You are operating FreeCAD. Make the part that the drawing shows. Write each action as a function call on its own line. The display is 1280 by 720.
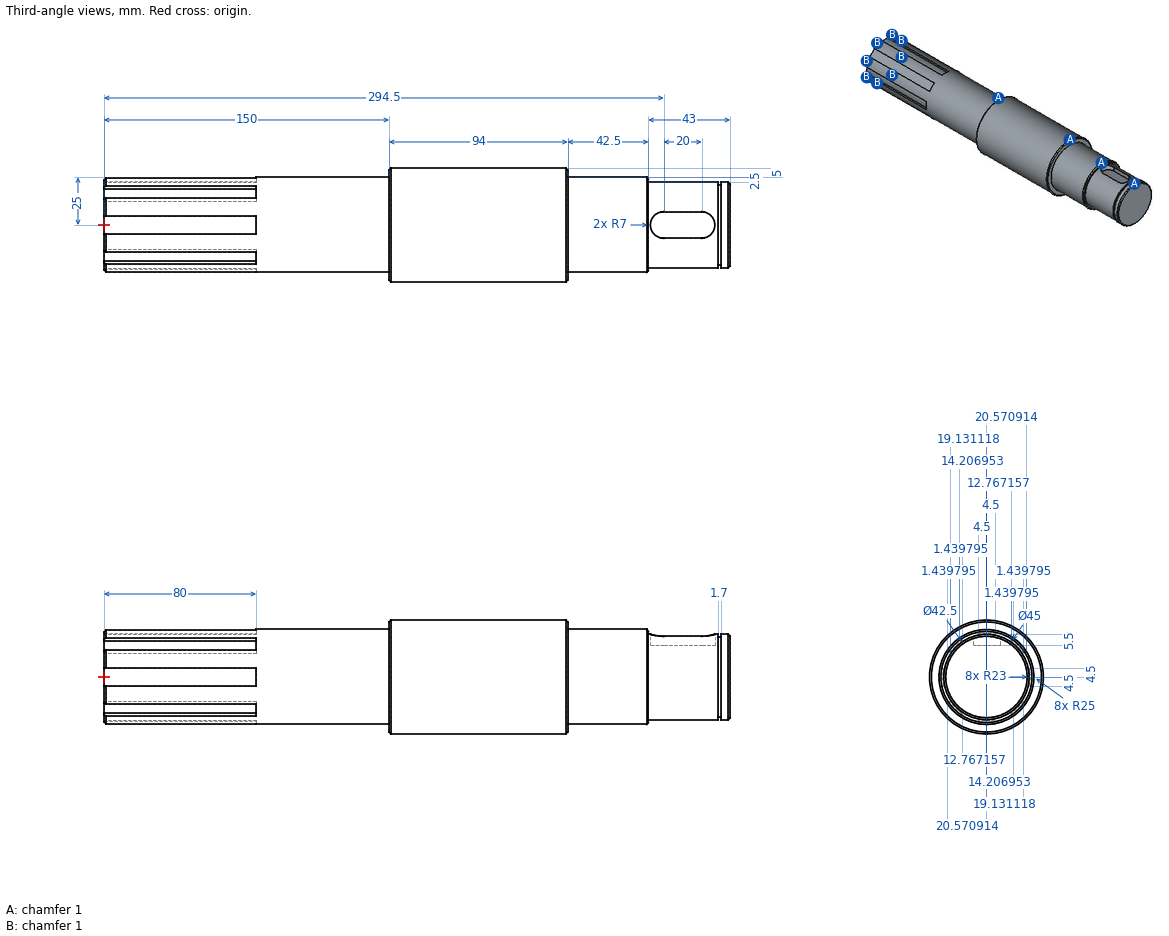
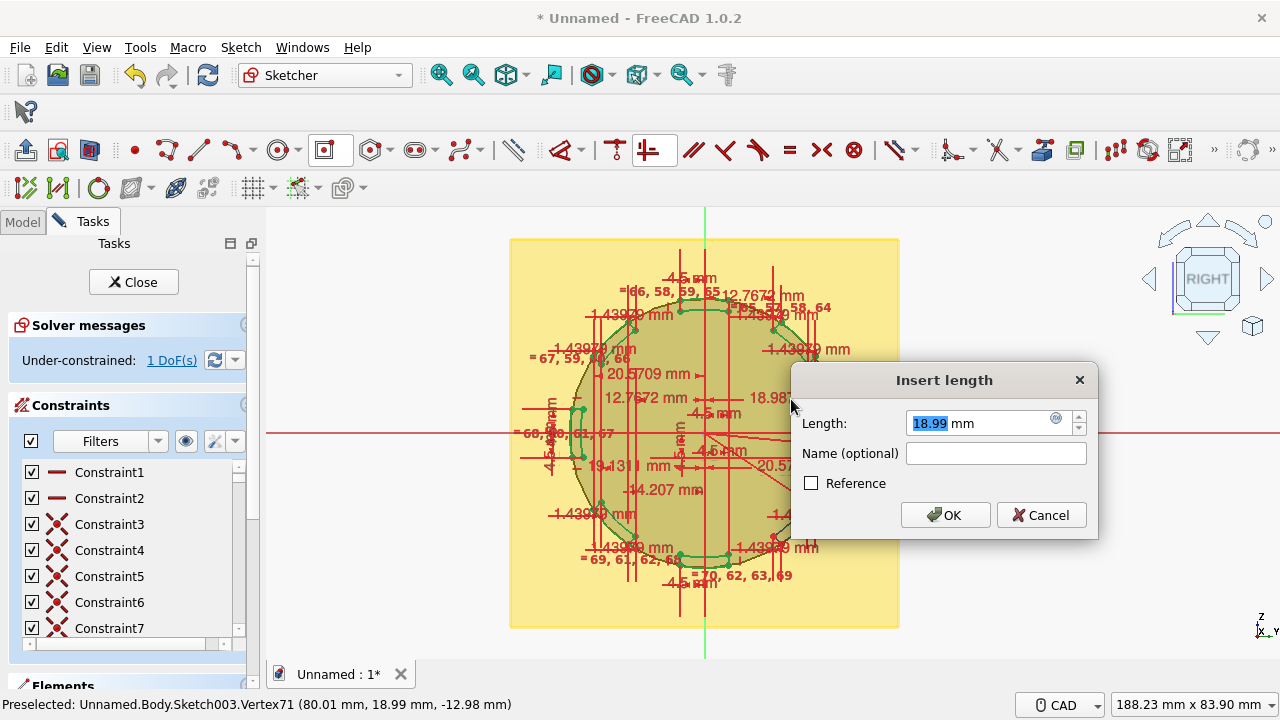
text(19.131118)
key(Return)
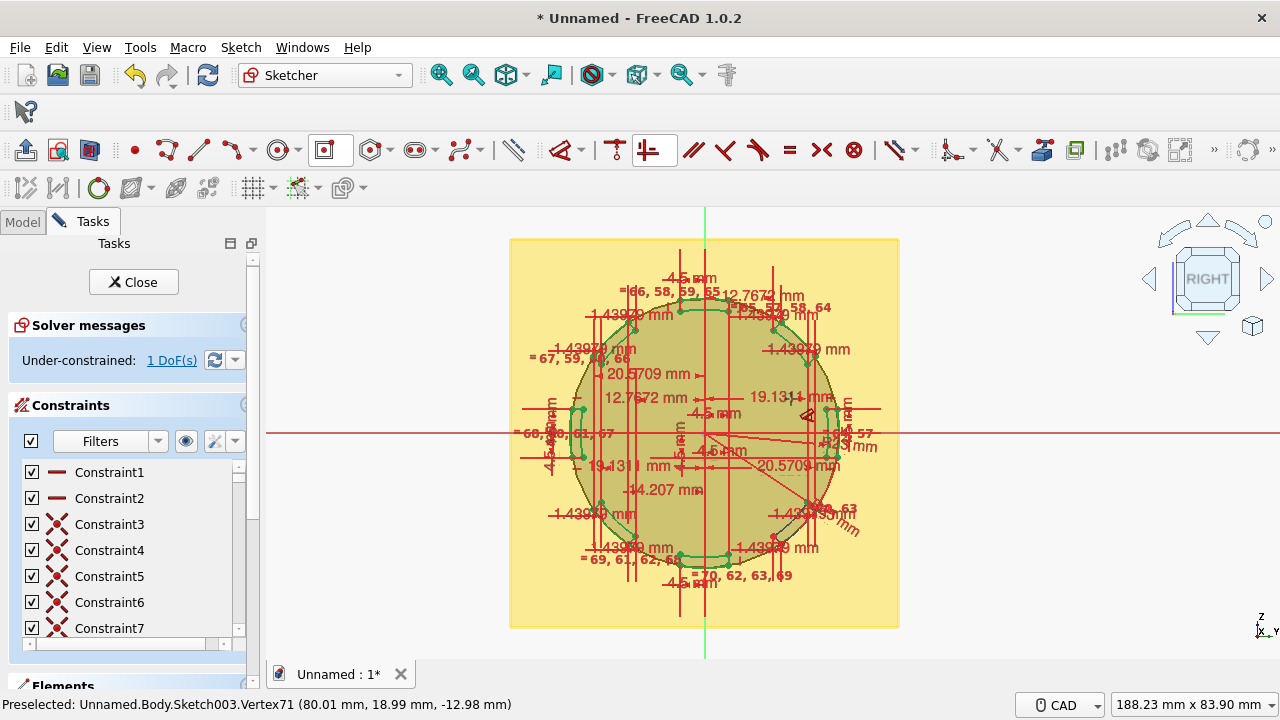
click(781, 544)
click(770, 578)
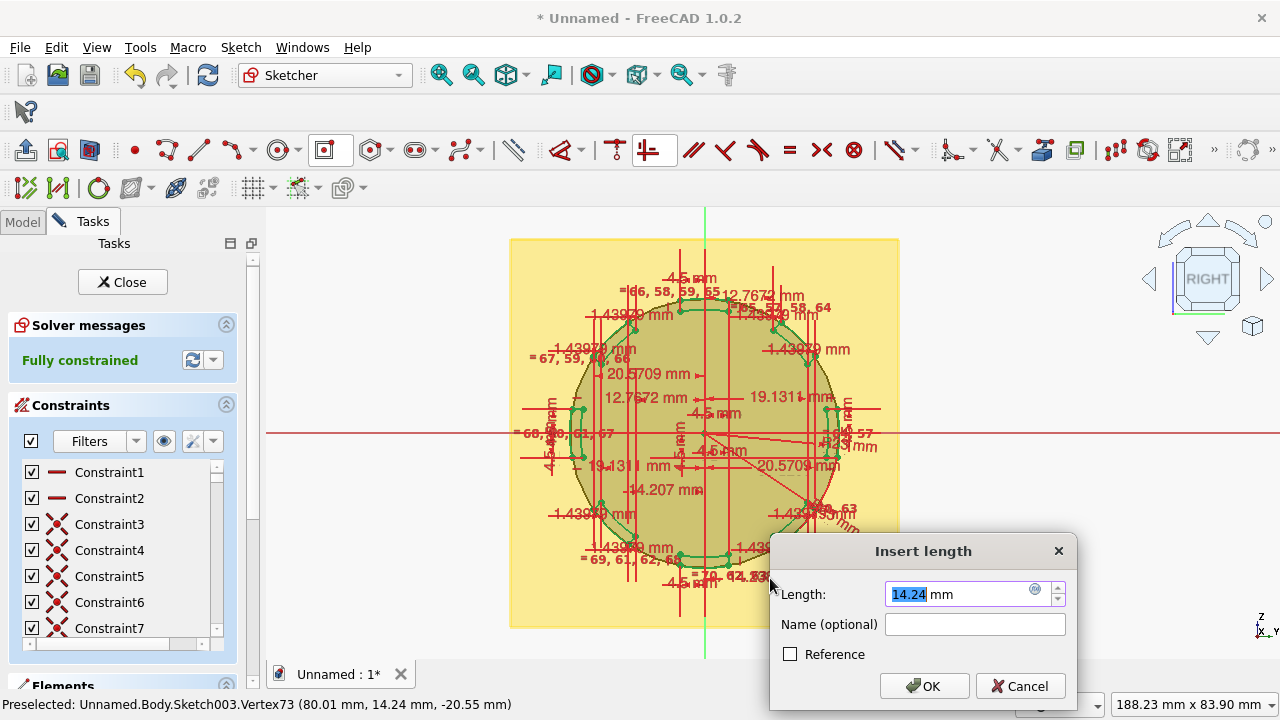
text(14.206953)
key(Return)
key(Escape)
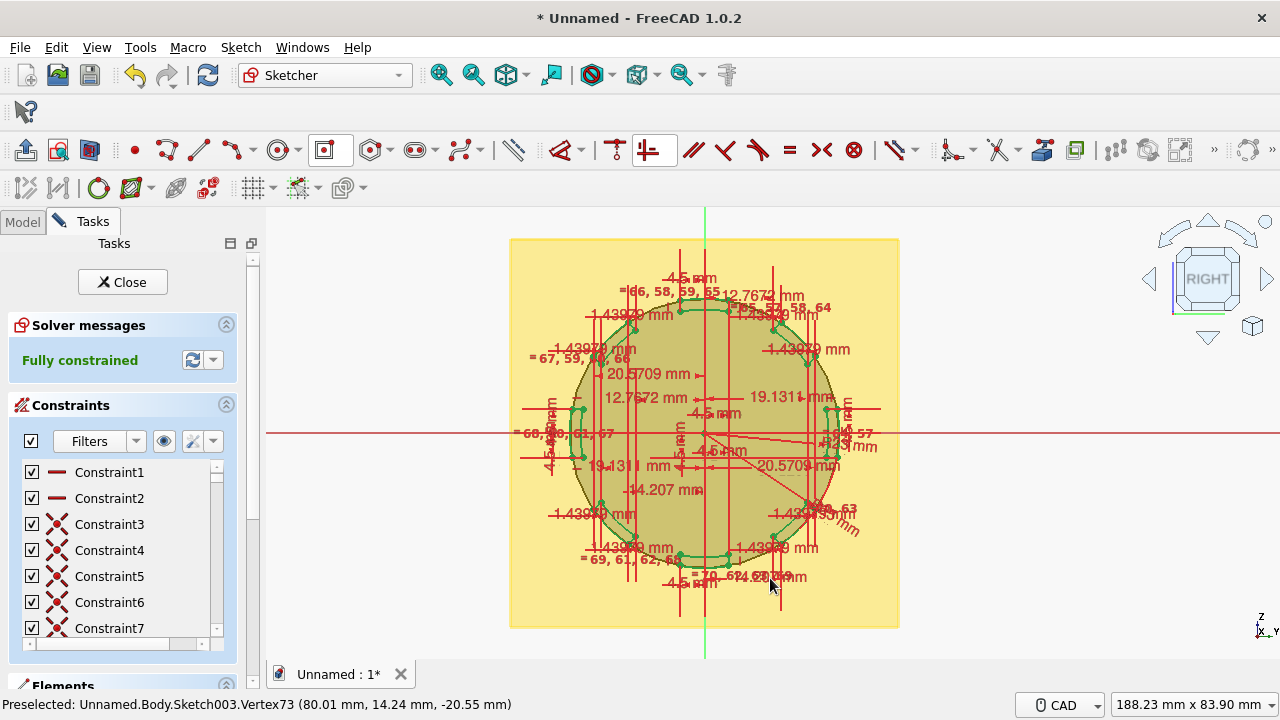
click(123, 282)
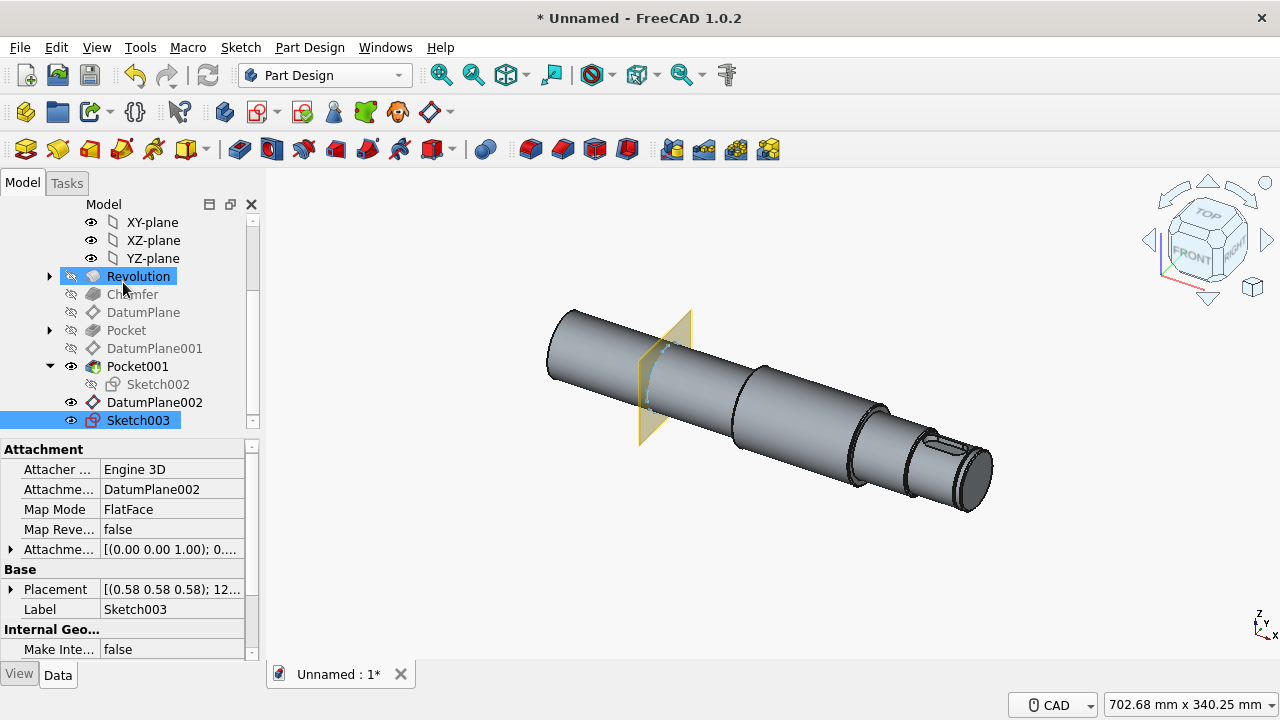
click(240, 150)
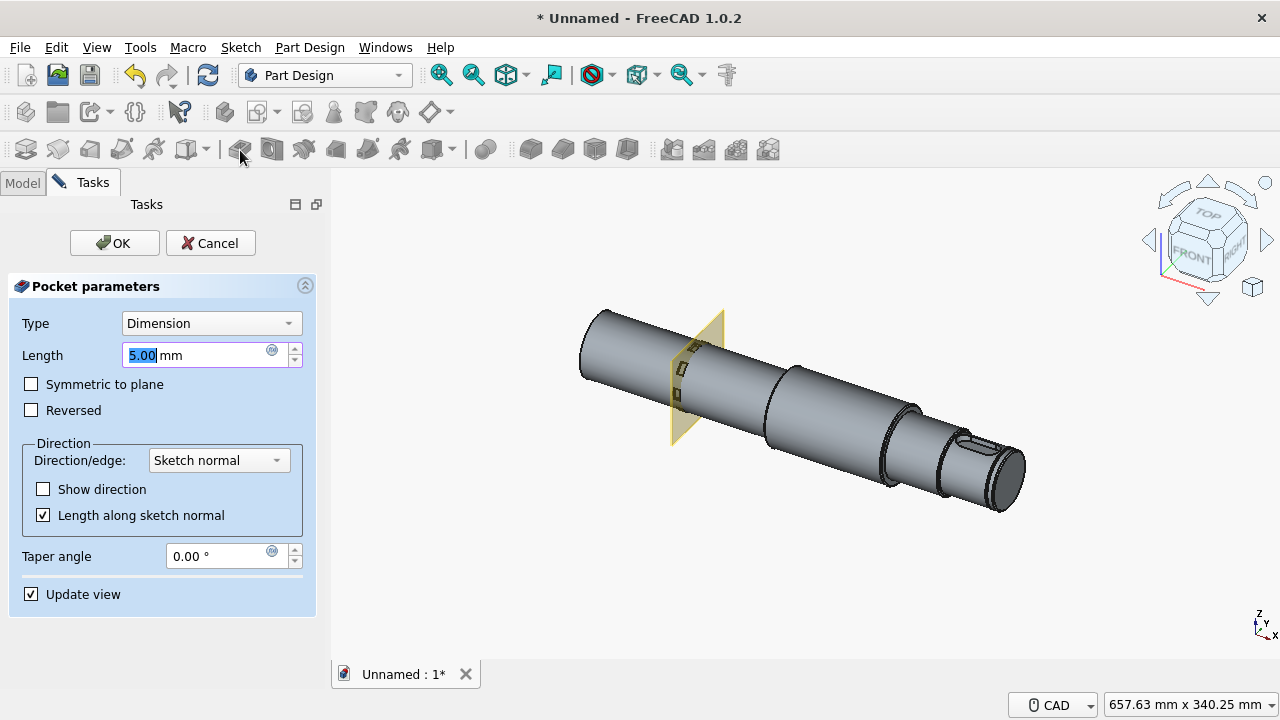
text(80)
key(Tab)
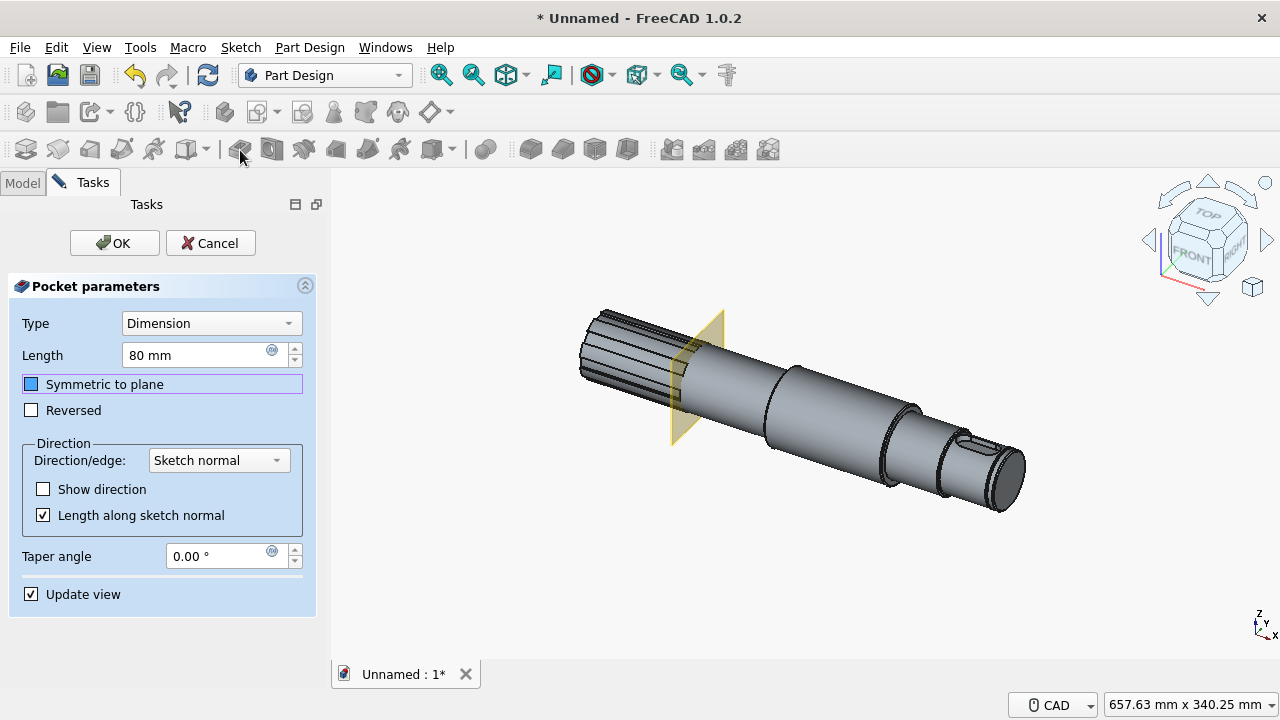
click(115, 243)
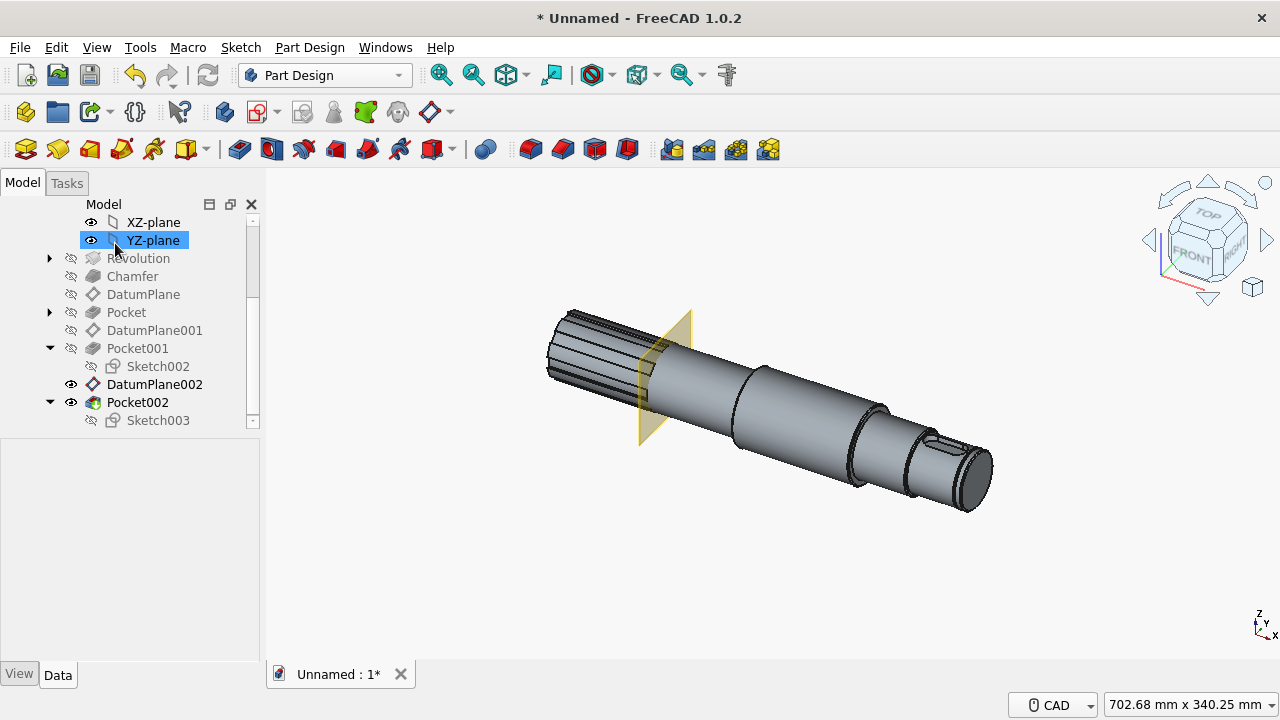
click(116, 384)
key(space)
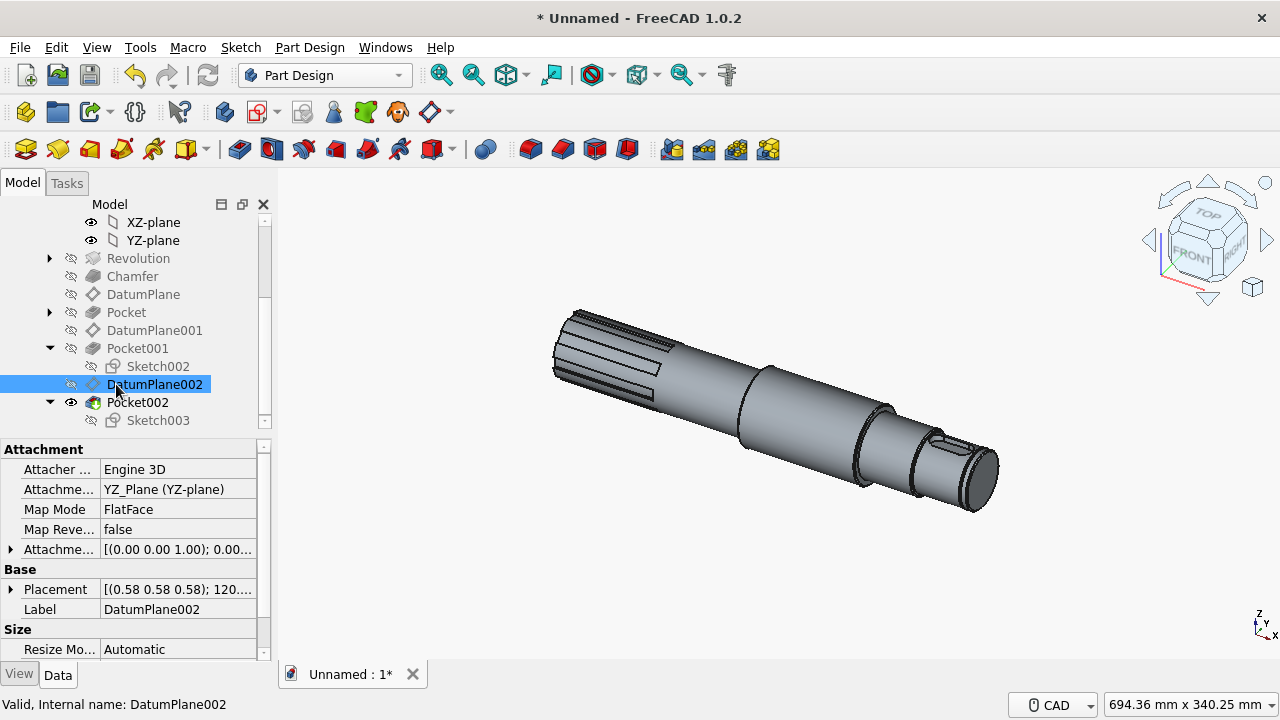
click(564, 323)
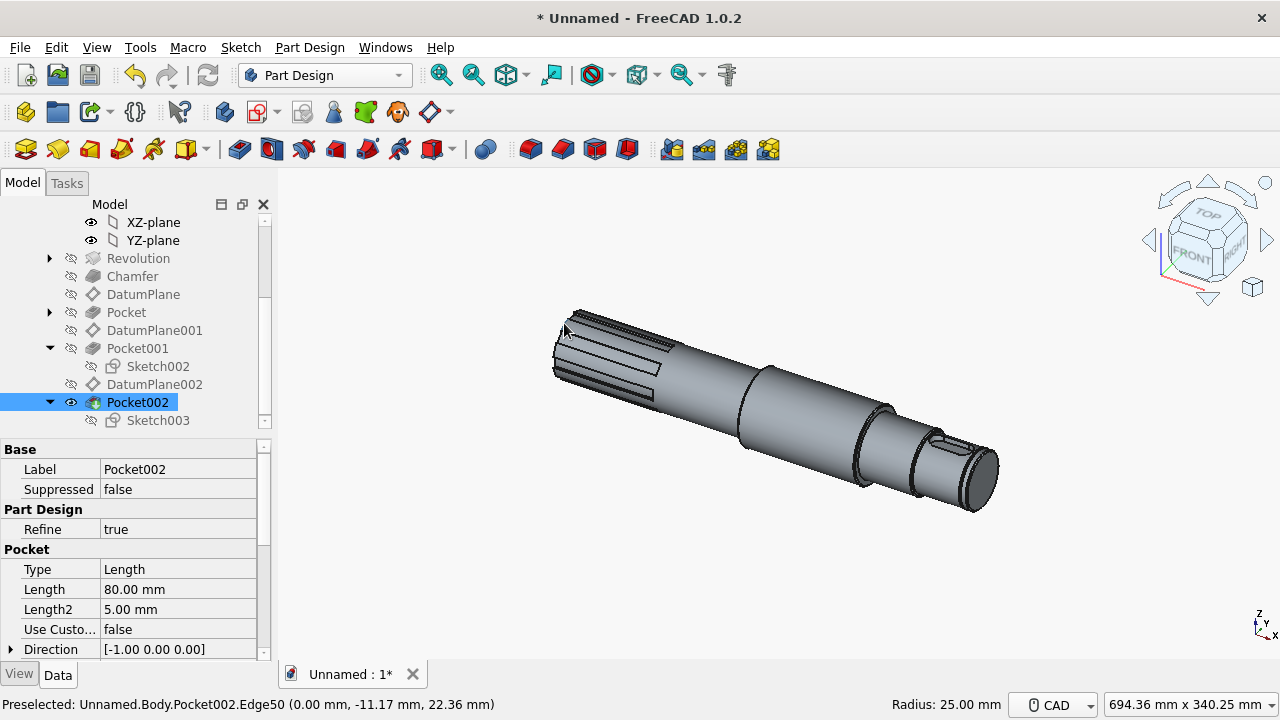
click(554, 350, ctrl)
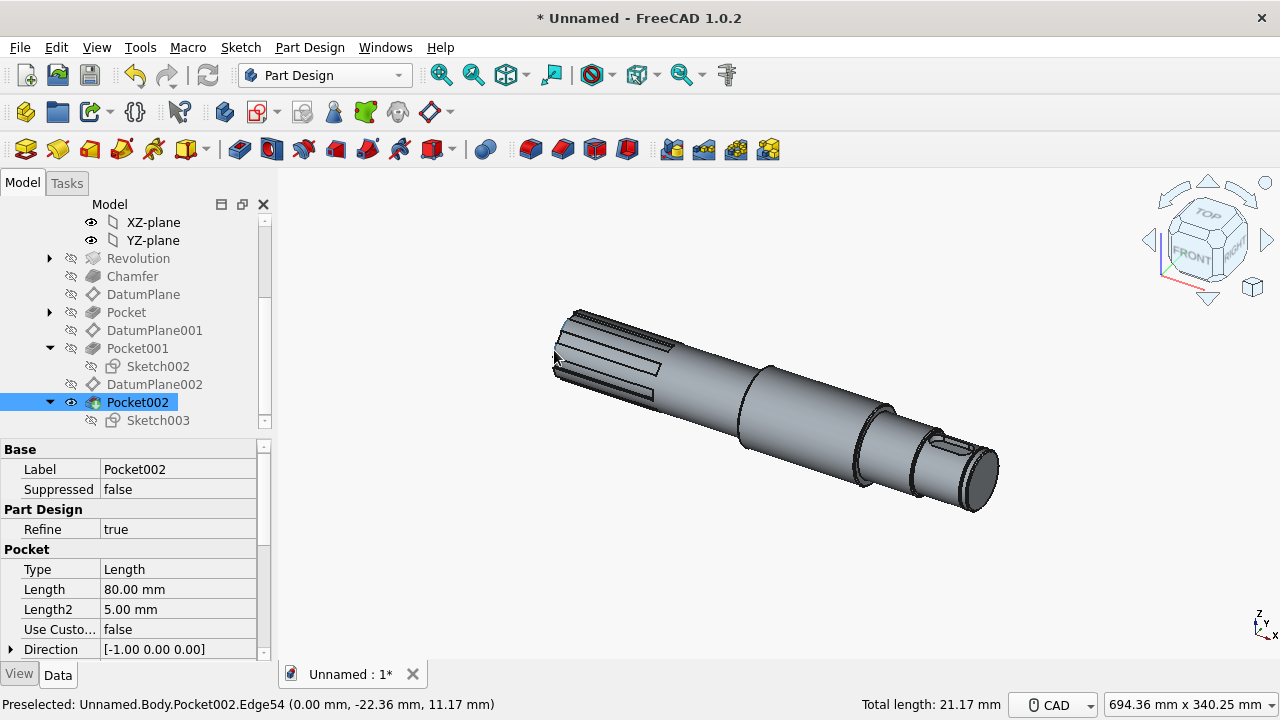
scroll(588, 316, up, 5)